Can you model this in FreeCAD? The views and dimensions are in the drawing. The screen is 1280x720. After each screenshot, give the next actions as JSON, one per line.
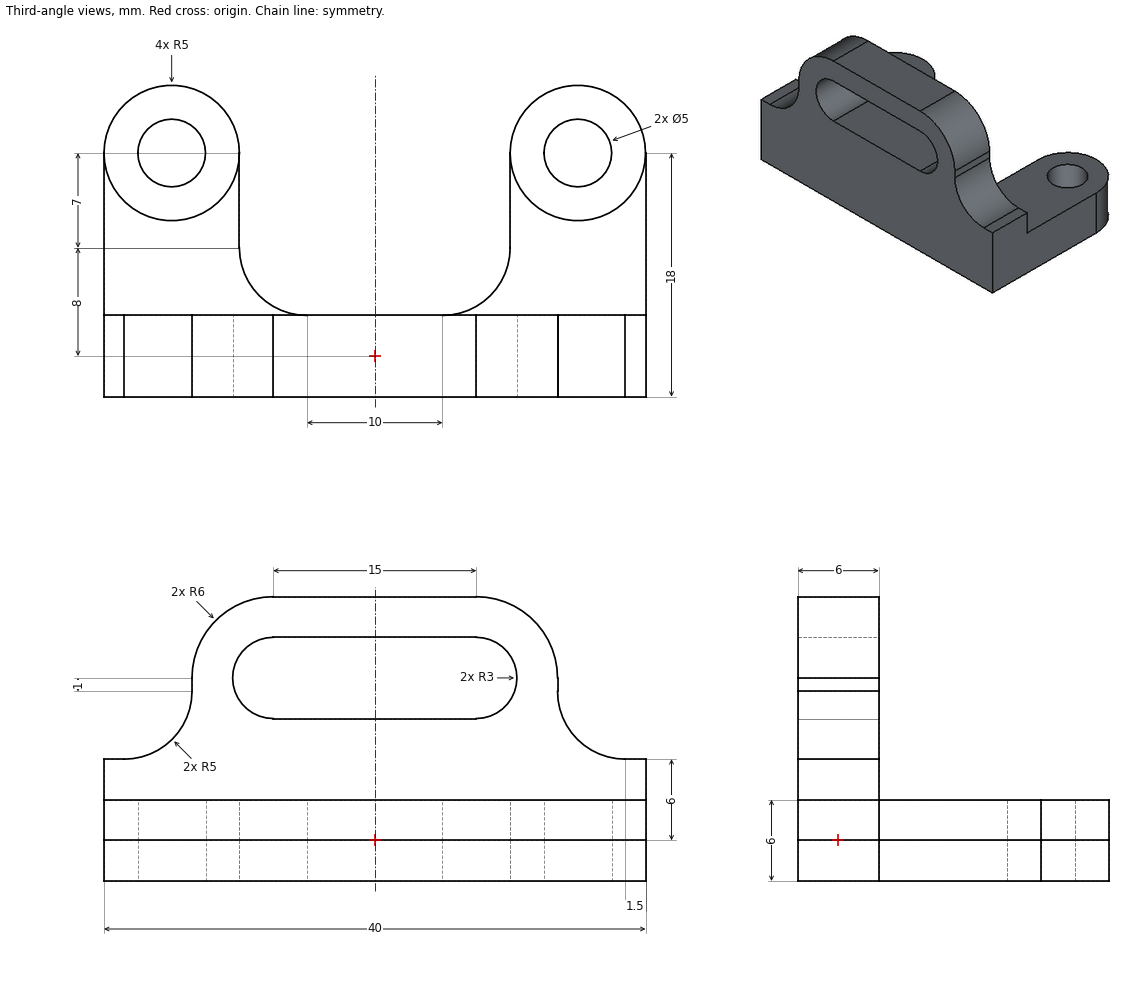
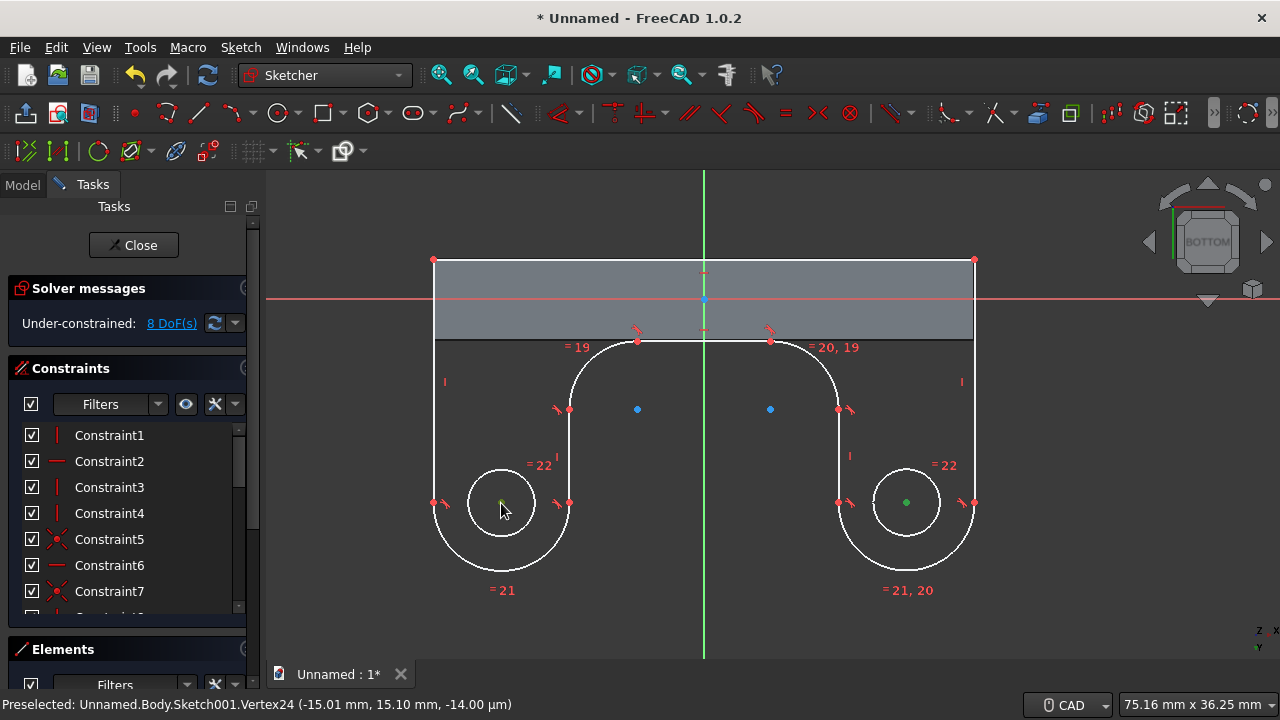
{"action": "left_click", "coordinate": [704, 600]}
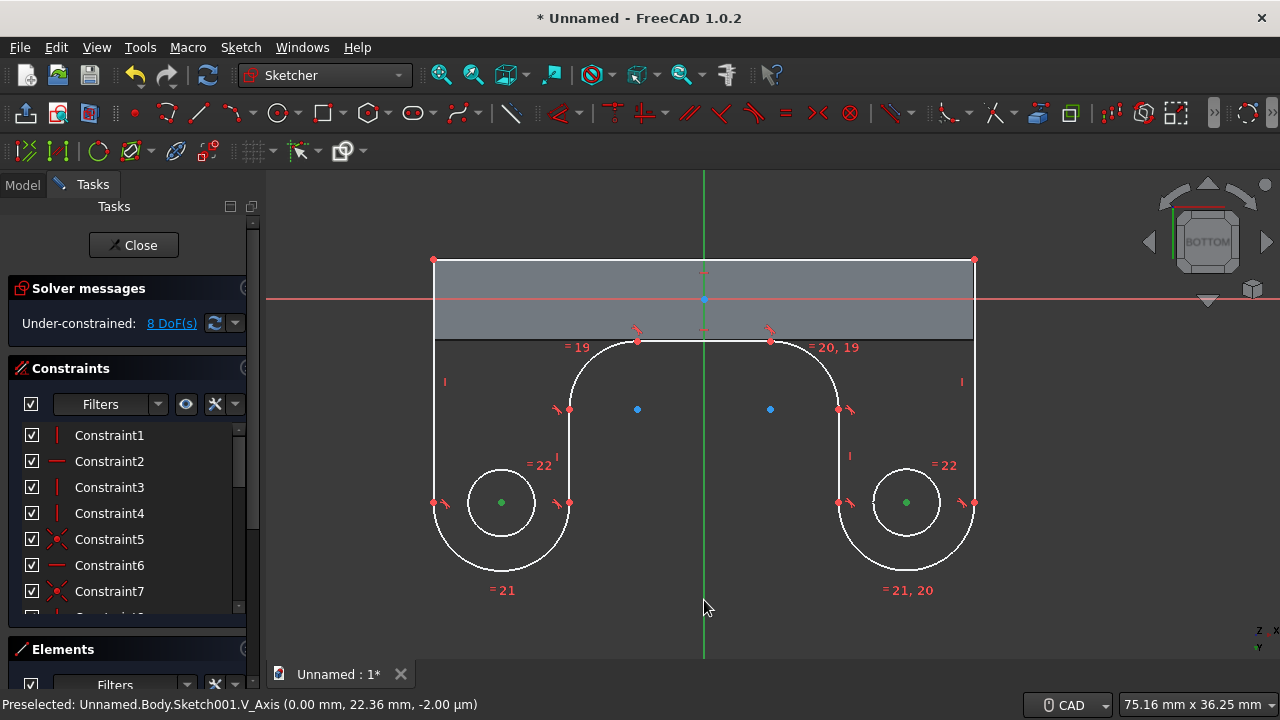
{"action": "left_click", "coordinate": [818, 114]}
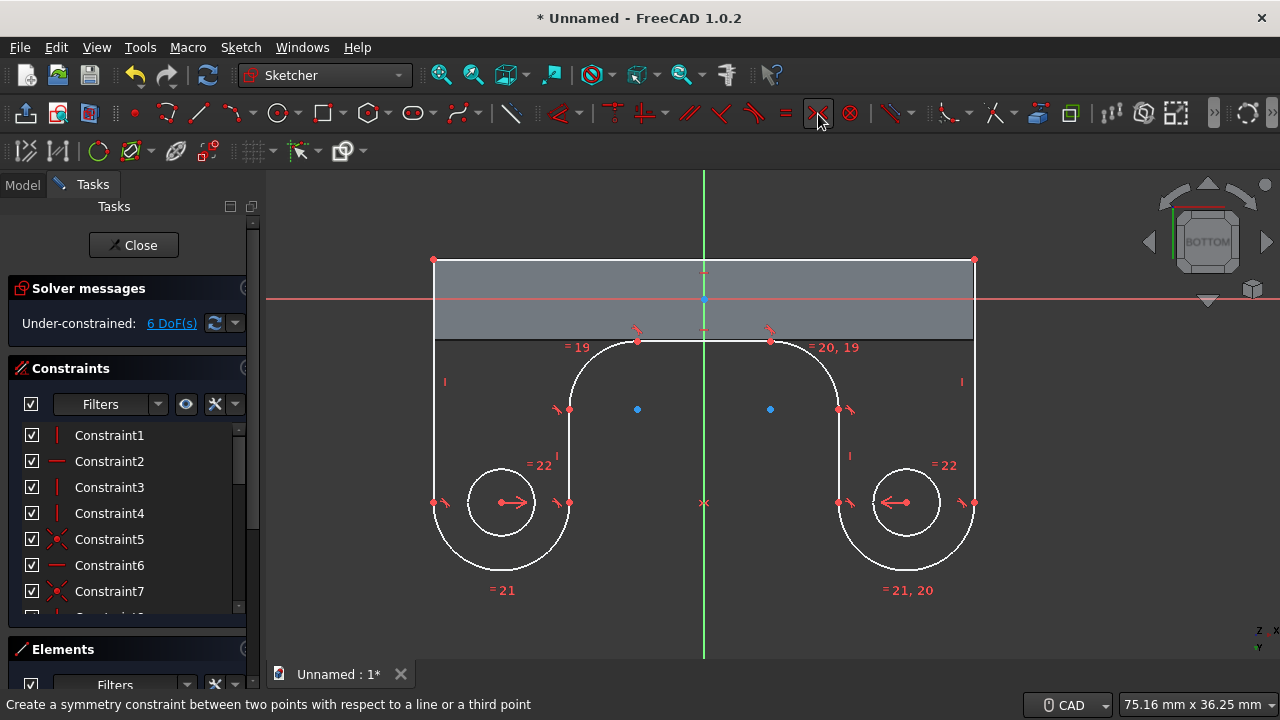
{"action": "key", "text": "d"}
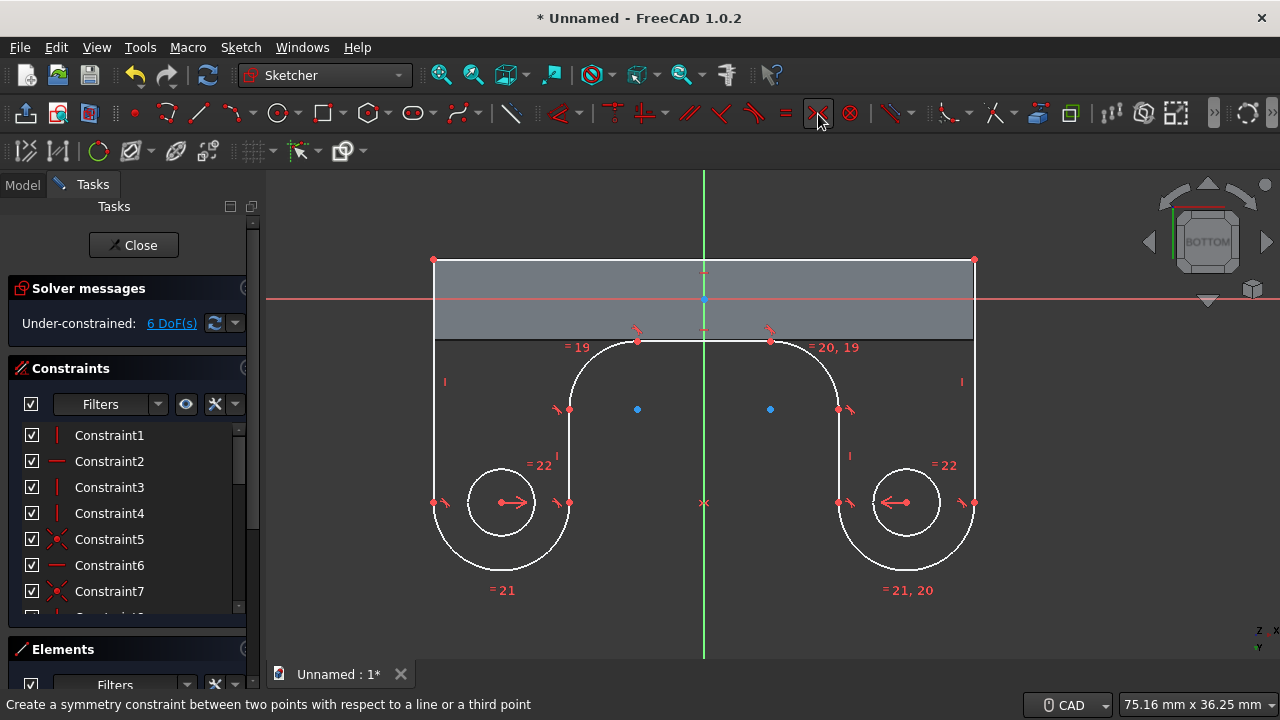
{"action": "left_click", "coordinate": [607, 349]}
{"action": "left_click", "coordinate": [593, 320]}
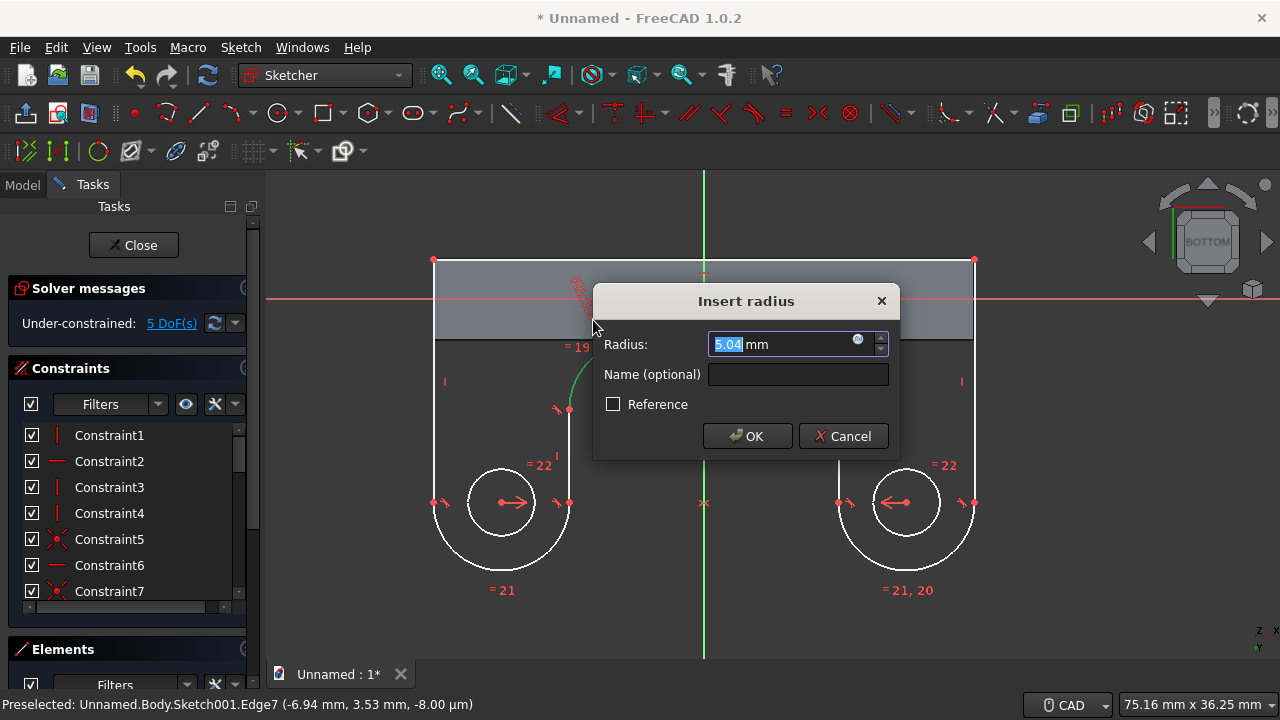
{"action": "type", "text": "5"}
{"action": "key", "text": "Return"}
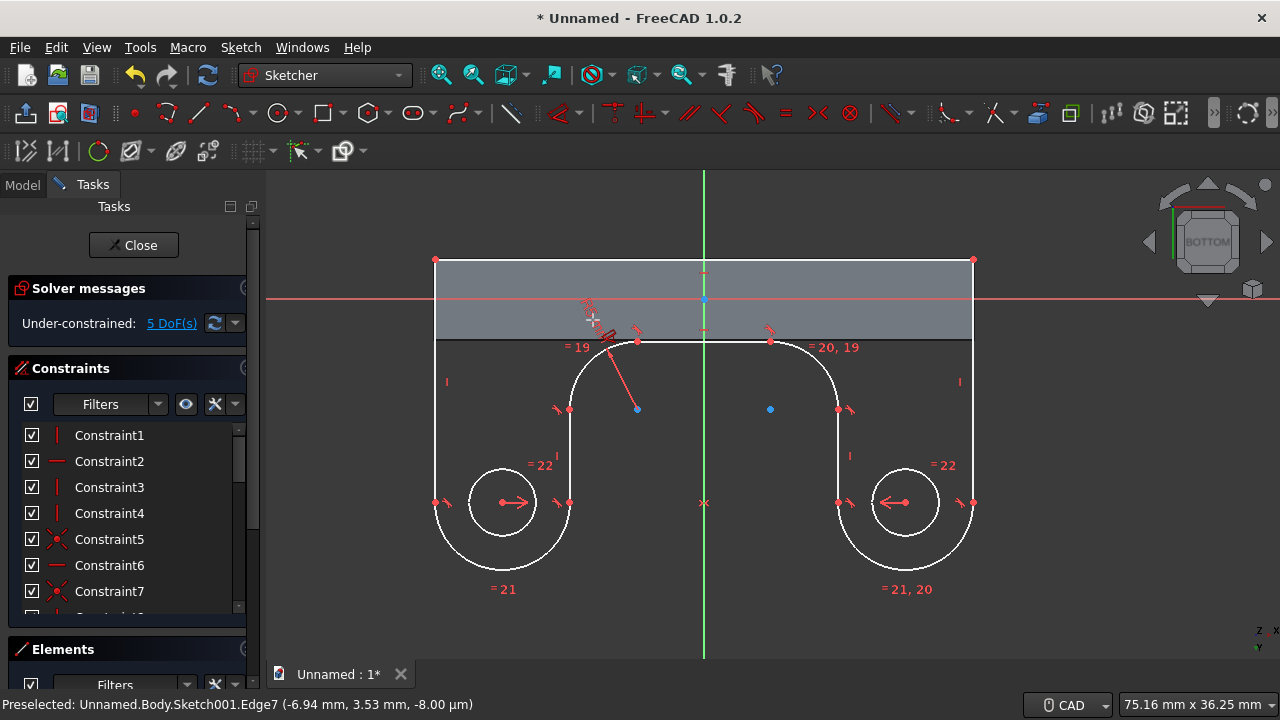
{"action": "left_click", "coordinate": [929, 479]}
{"action": "left_click", "coordinate": [952, 456]}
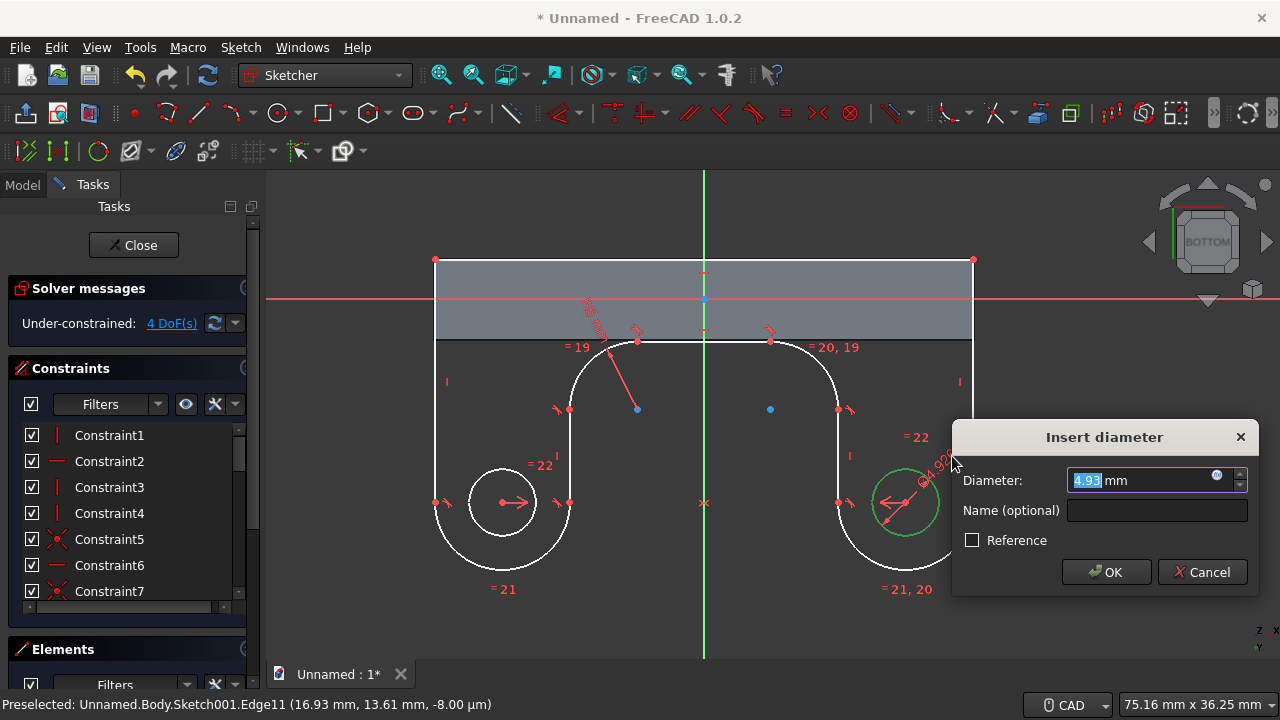
{"action": "type", "text": "5"}
{"action": "key", "text": "Return"}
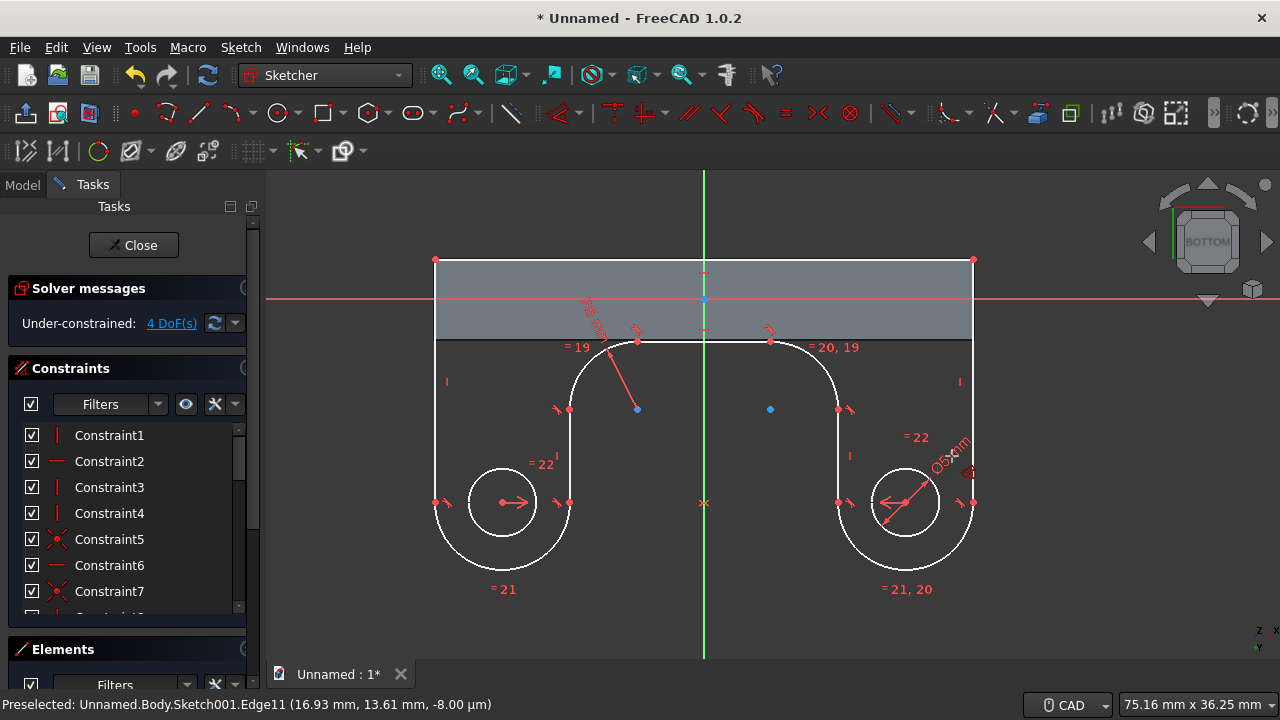
{"action": "left_click", "coordinate": [570, 475]}
{"action": "left_click", "coordinate": [536, 456]}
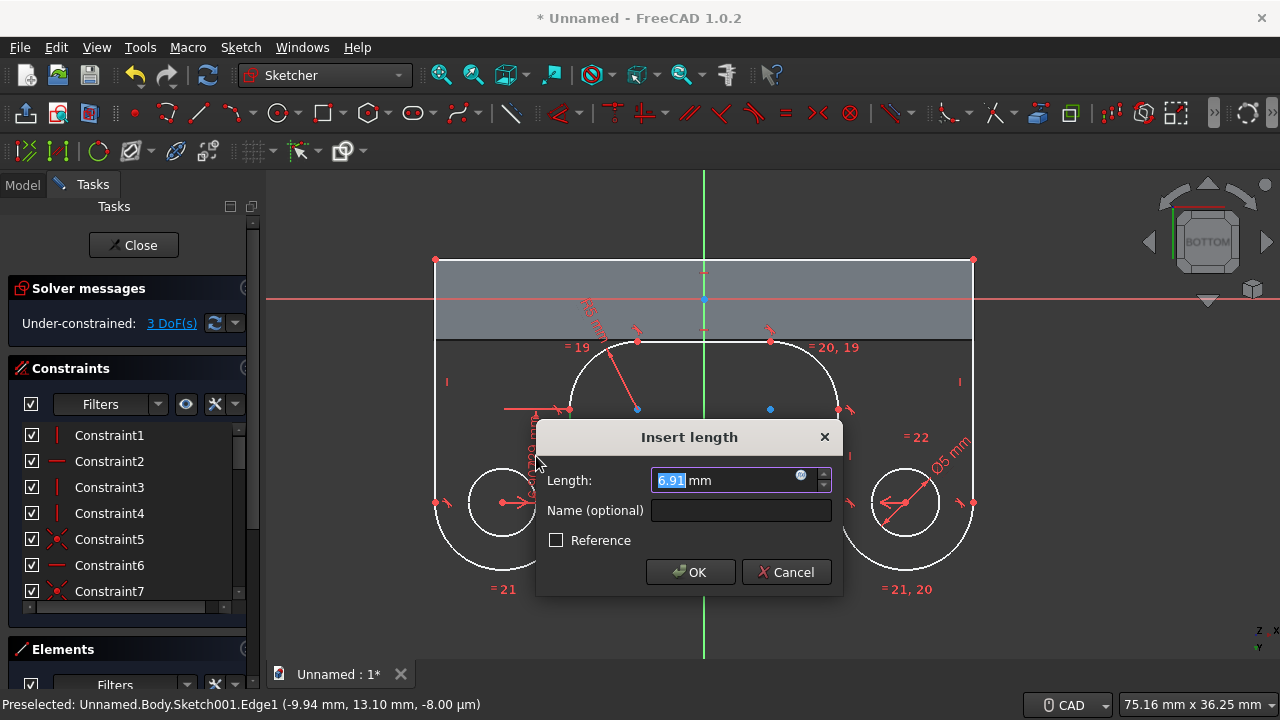
{"action": "type", "text": "7"}
{"action": "key", "text": "Return"}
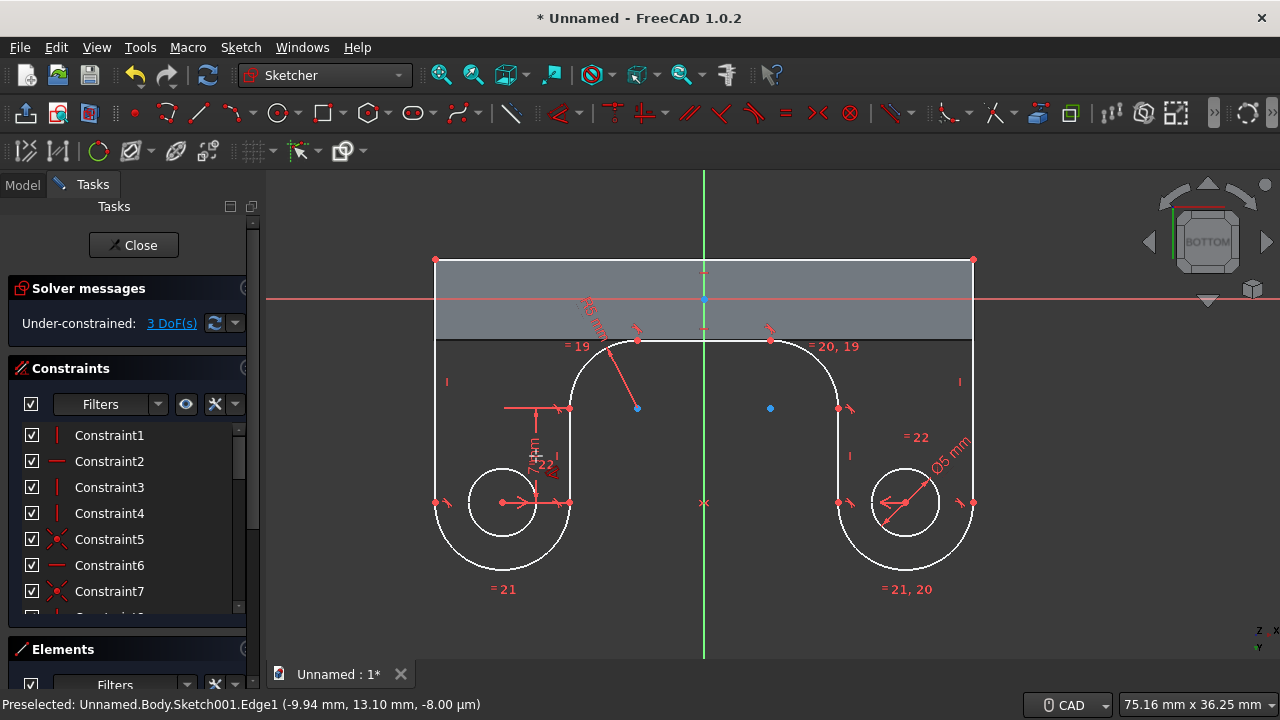
{"action": "left_click", "coordinate": [677, 341]}
{"action": "left_click", "coordinate": [673, 375]}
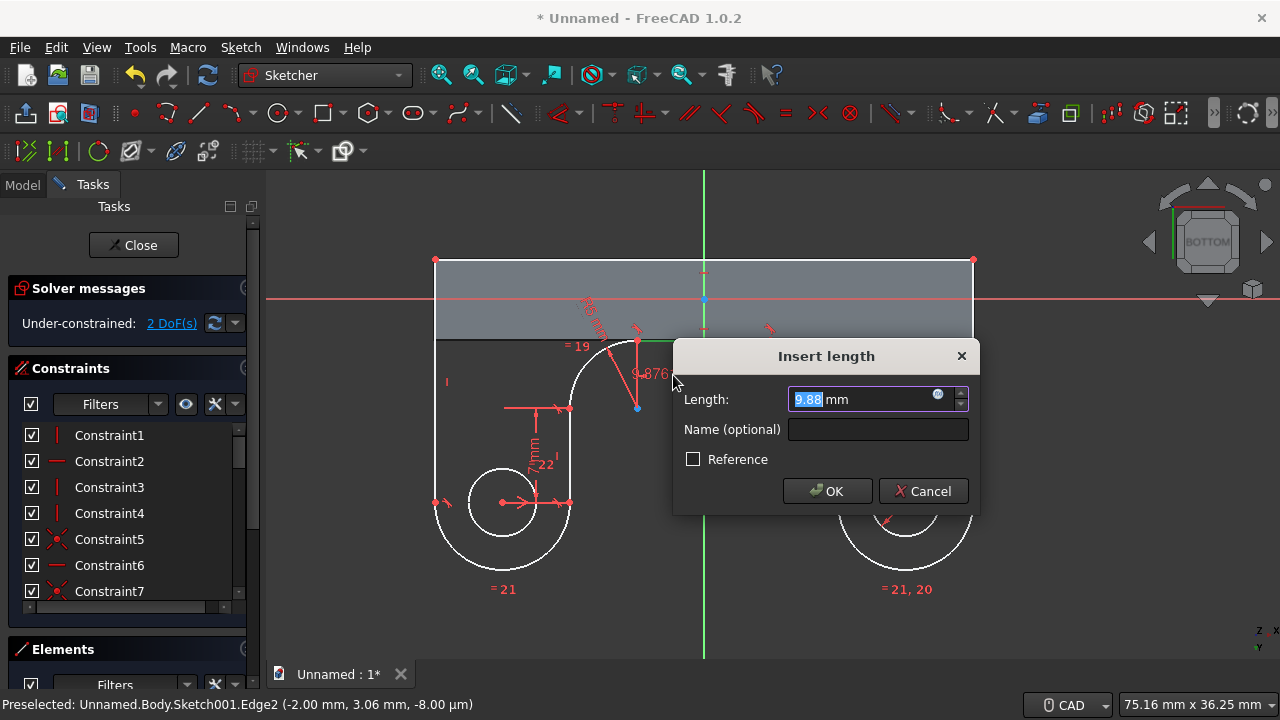
{"action": "type", "text": "10"}
{"action": "key", "text": "Return"}